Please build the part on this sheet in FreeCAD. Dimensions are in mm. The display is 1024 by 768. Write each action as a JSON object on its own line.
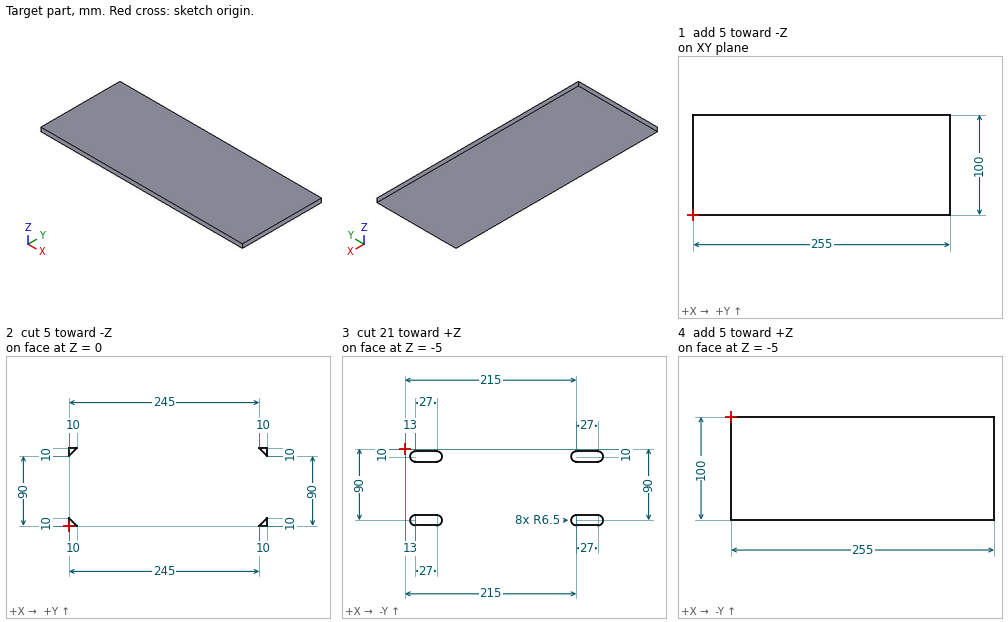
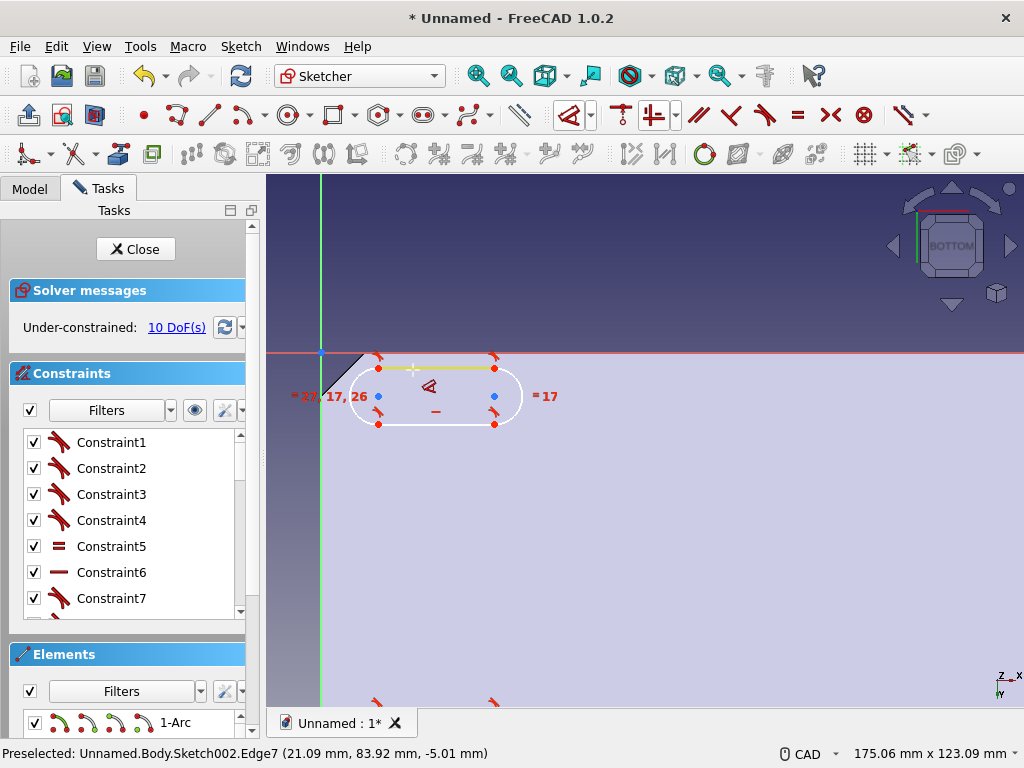
{"action": "left_click", "coordinate": [413, 368]}
{"action": "left_click", "coordinate": [436, 334]}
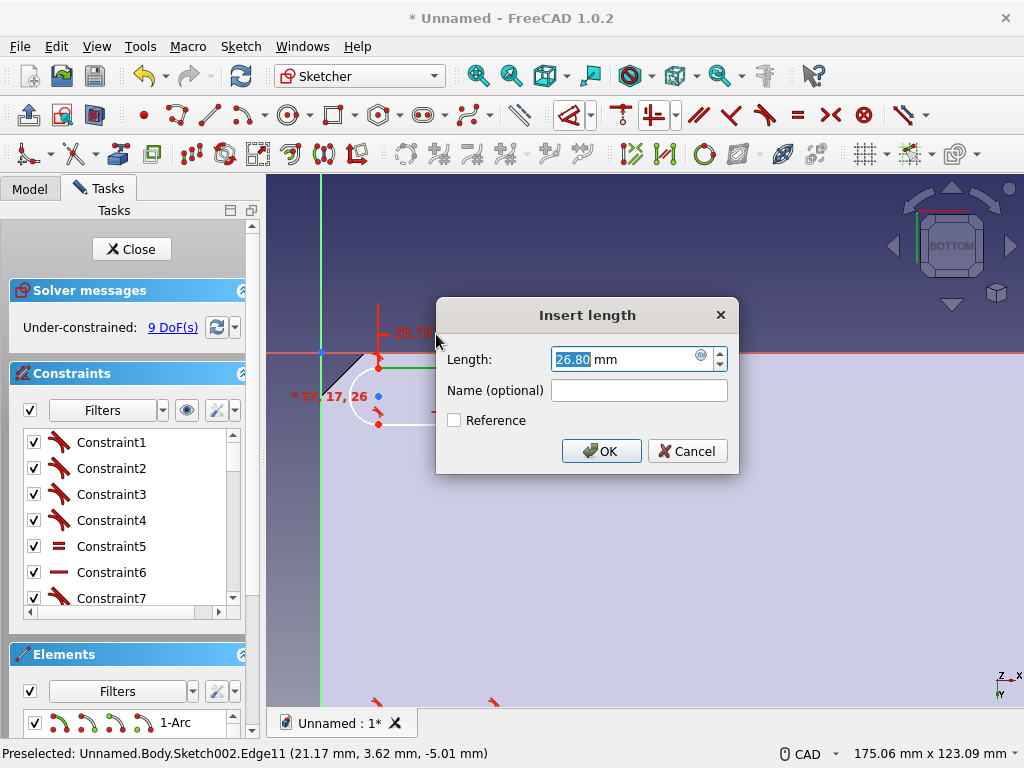
{"action": "type", "text": "27"}
{"action": "key", "text": "Return"}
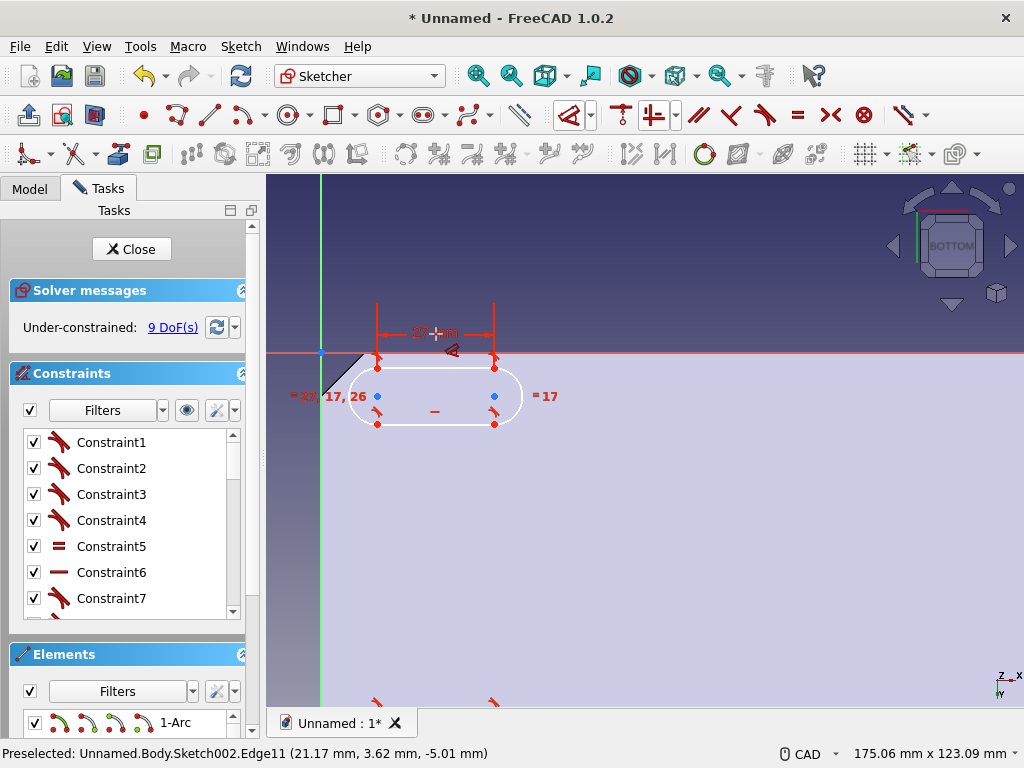
{"action": "scroll", "coordinate": [412, 370], "scroll_direction": "down", "scroll_amount": 5}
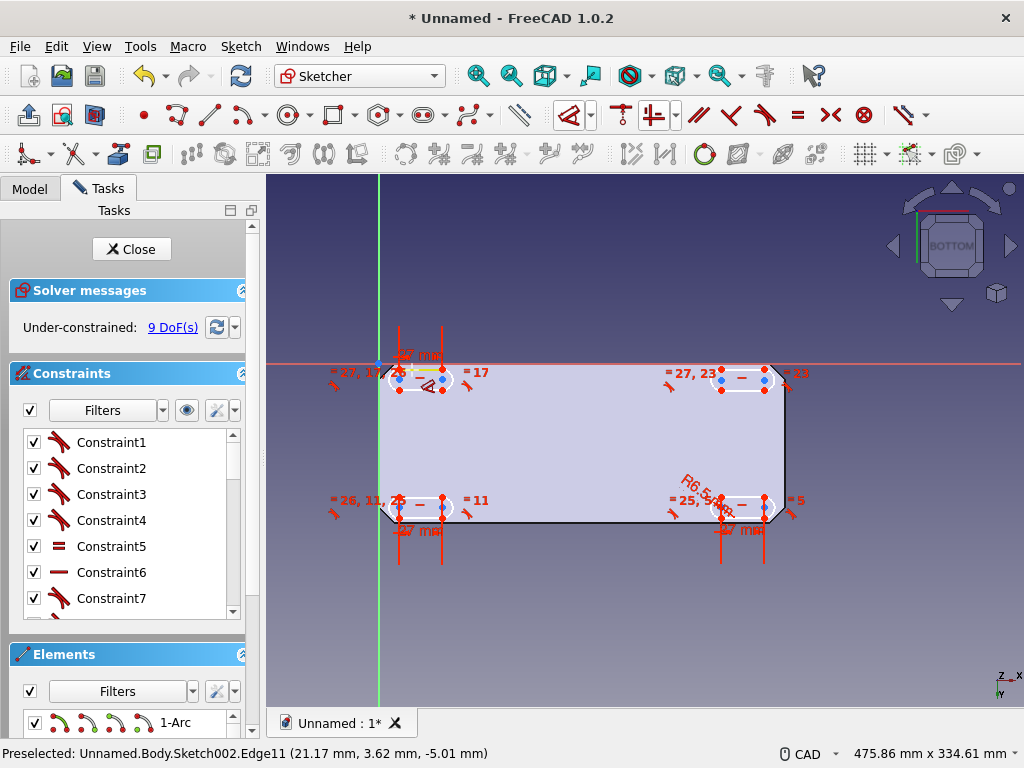
{"action": "scroll", "coordinate": [734, 370], "scroll_direction": "up", "scroll_amount": 5}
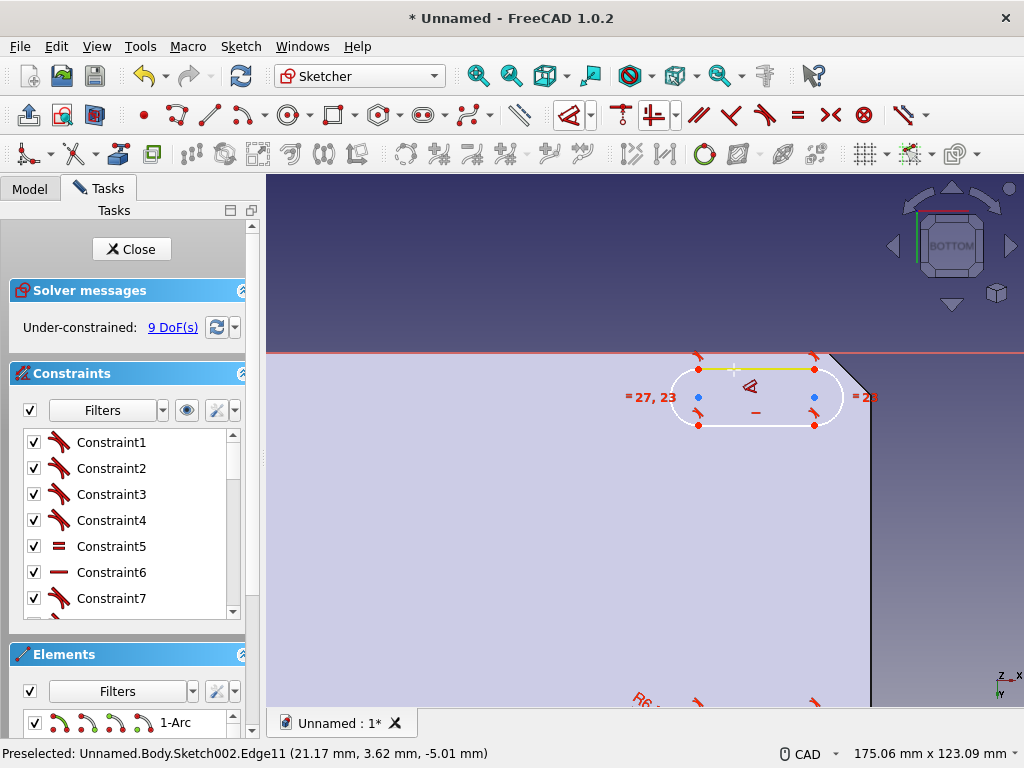
{"action": "left_click", "coordinate": [734, 369]}
{"action": "left_click", "coordinate": [757, 335]}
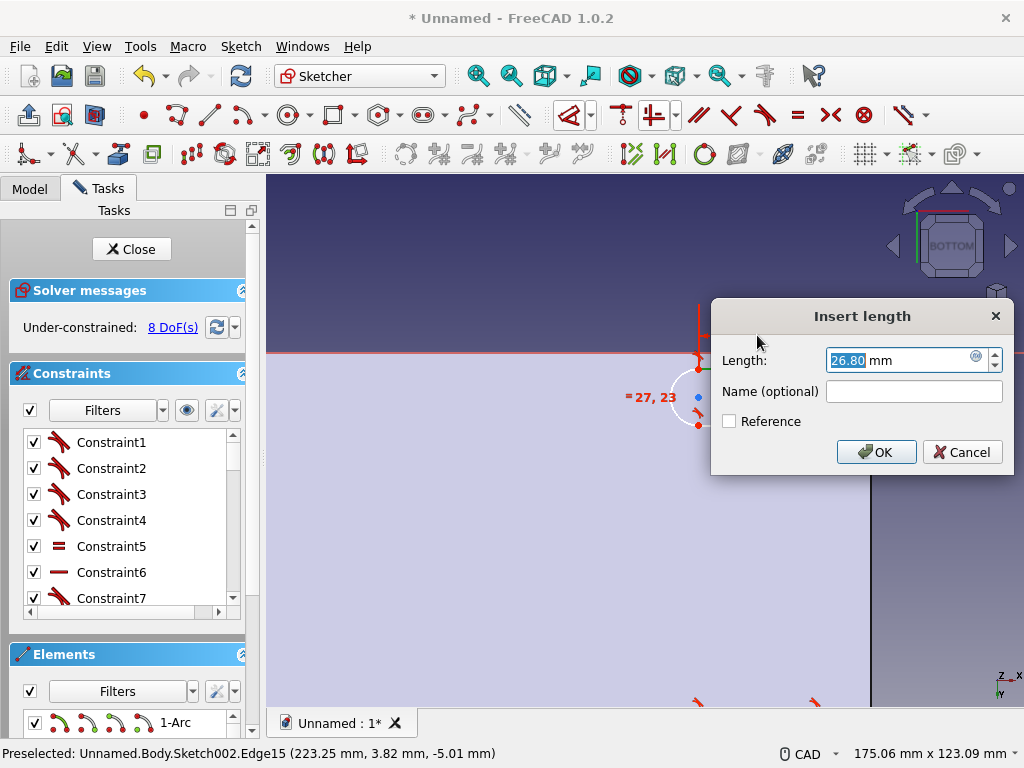
{"action": "type", "text": "27"}
{"action": "key", "text": "Return"}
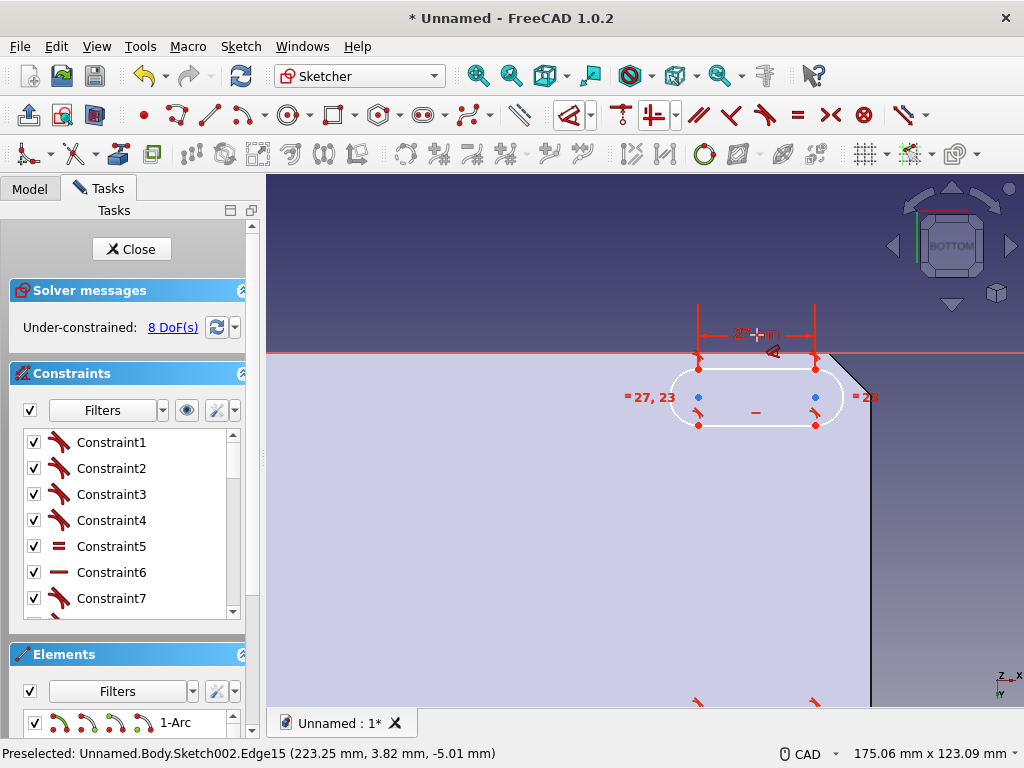
{"action": "scroll", "coordinate": [734, 370], "scroll_direction": "down", "scroll_amount": 5}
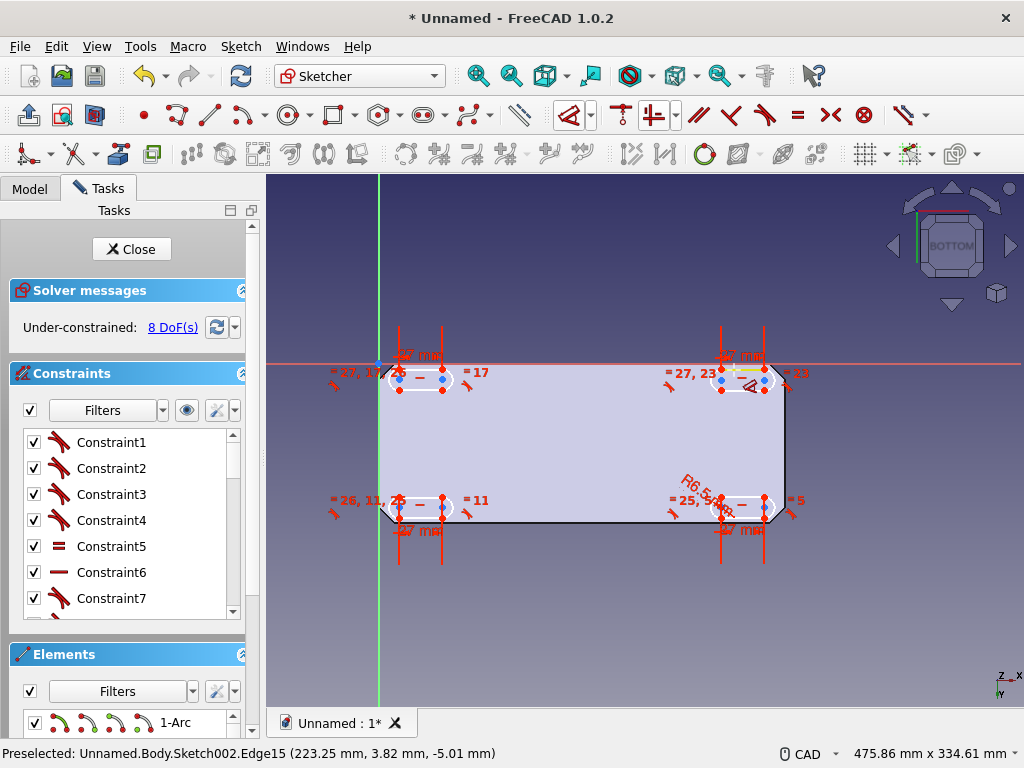
{"action": "scroll", "coordinate": [399, 498], "scroll_direction": "up", "scroll_amount": 4}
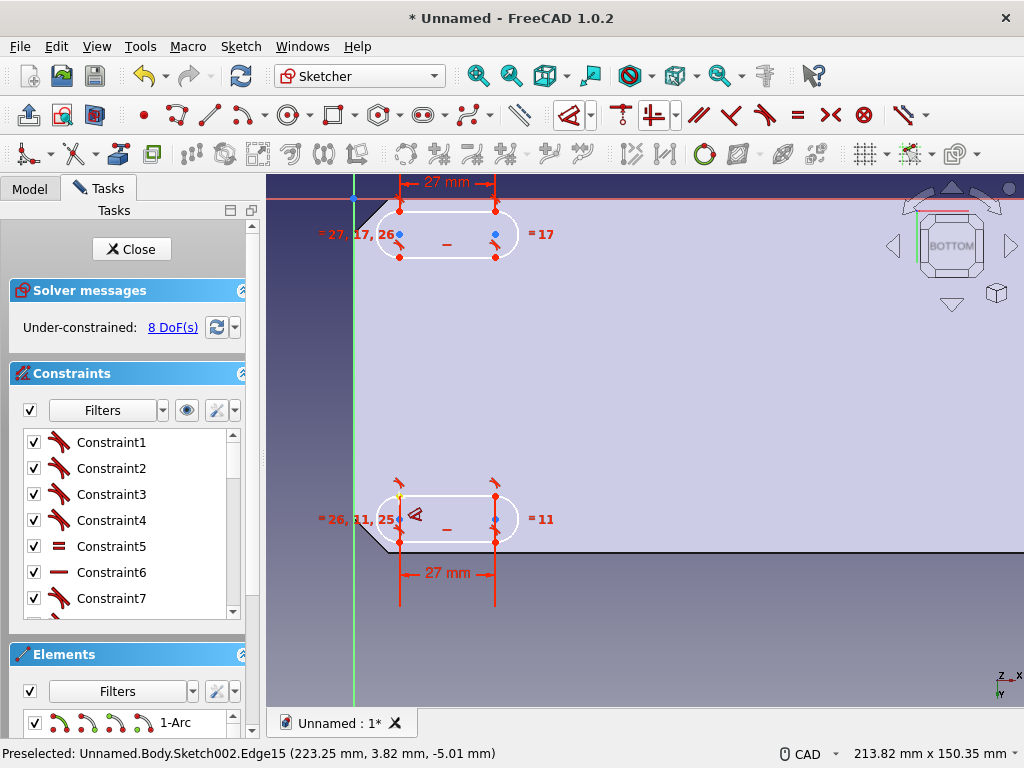
{"action": "left_click", "coordinate": [400, 496]}
{"action": "left_click", "coordinate": [377, 554]}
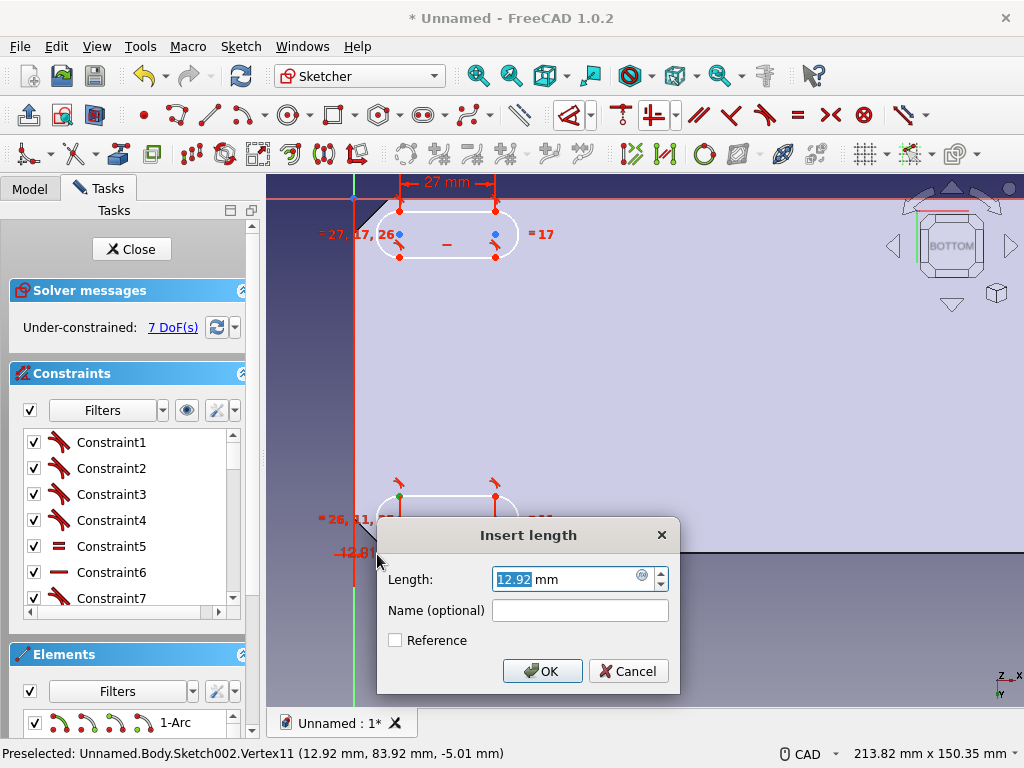
{"action": "type", "text": "13"}
{"action": "key", "text": "Return"}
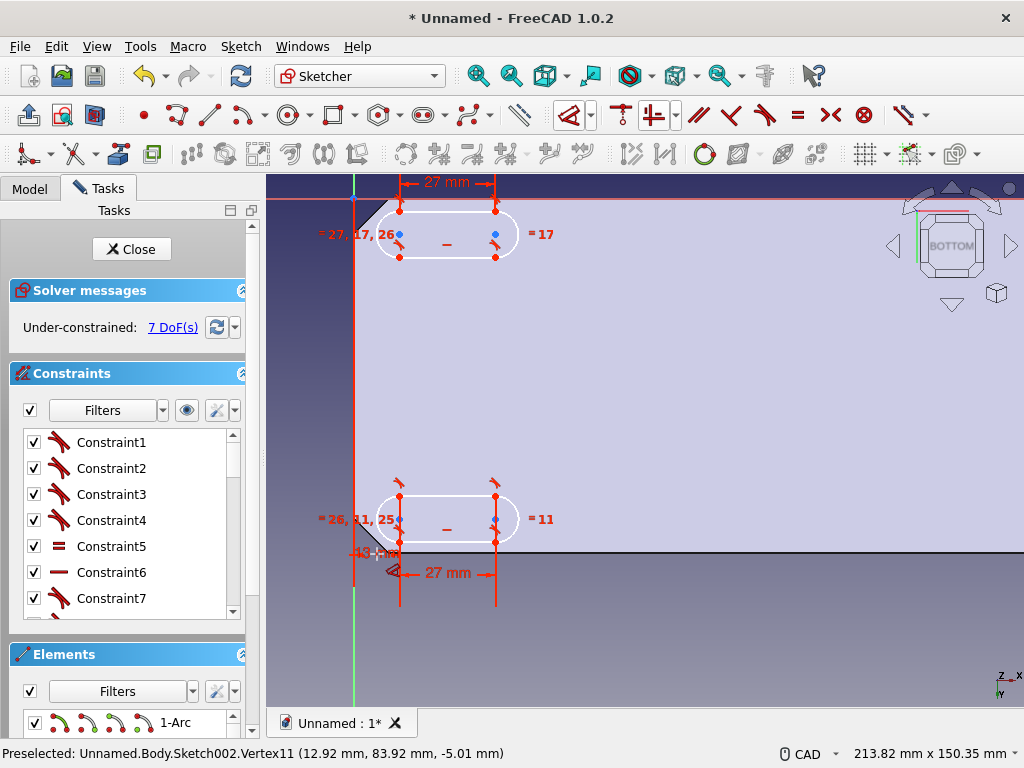
{"action": "left_click", "coordinate": [400, 212]}
{"action": "left_click", "coordinate": [377, 270]}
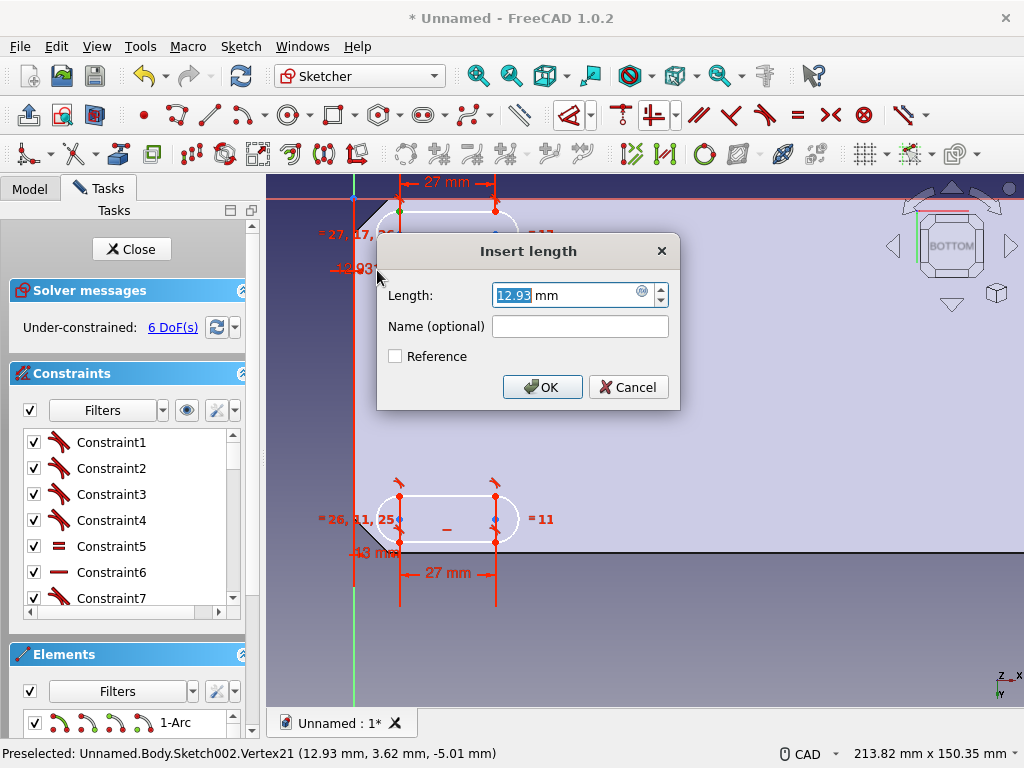
{"action": "type", "text": "13"}
{"action": "key", "text": "Return"}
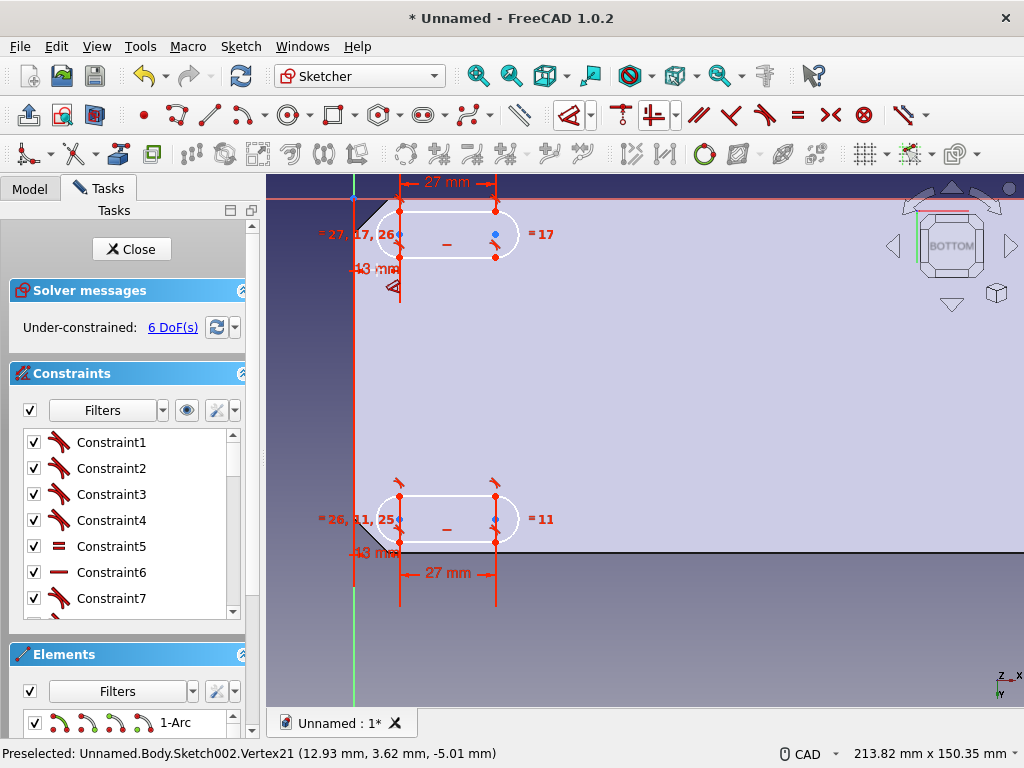
{"action": "scroll", "coordinate": [399, 498], "scroll_direction": "down", "scroll_amount": 4}